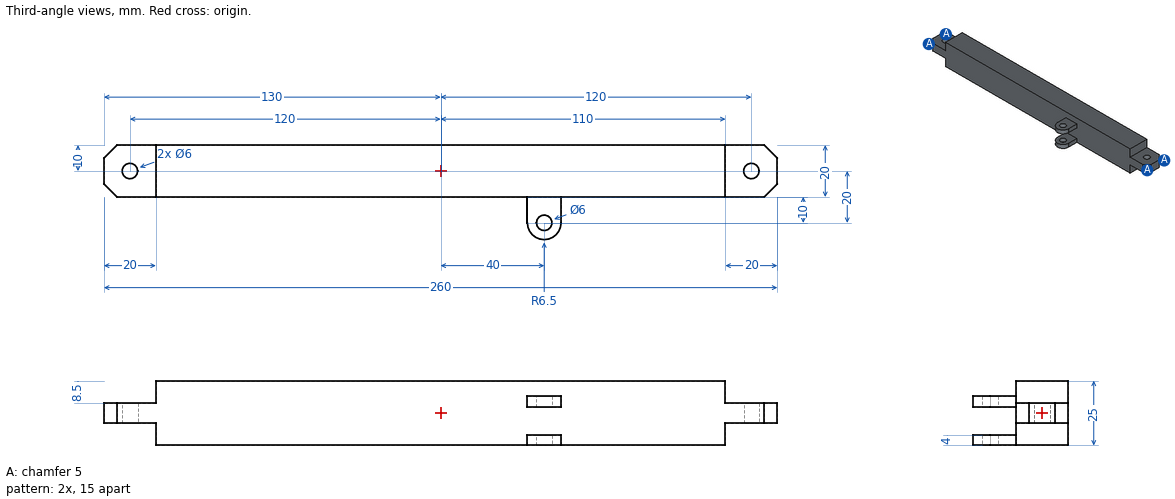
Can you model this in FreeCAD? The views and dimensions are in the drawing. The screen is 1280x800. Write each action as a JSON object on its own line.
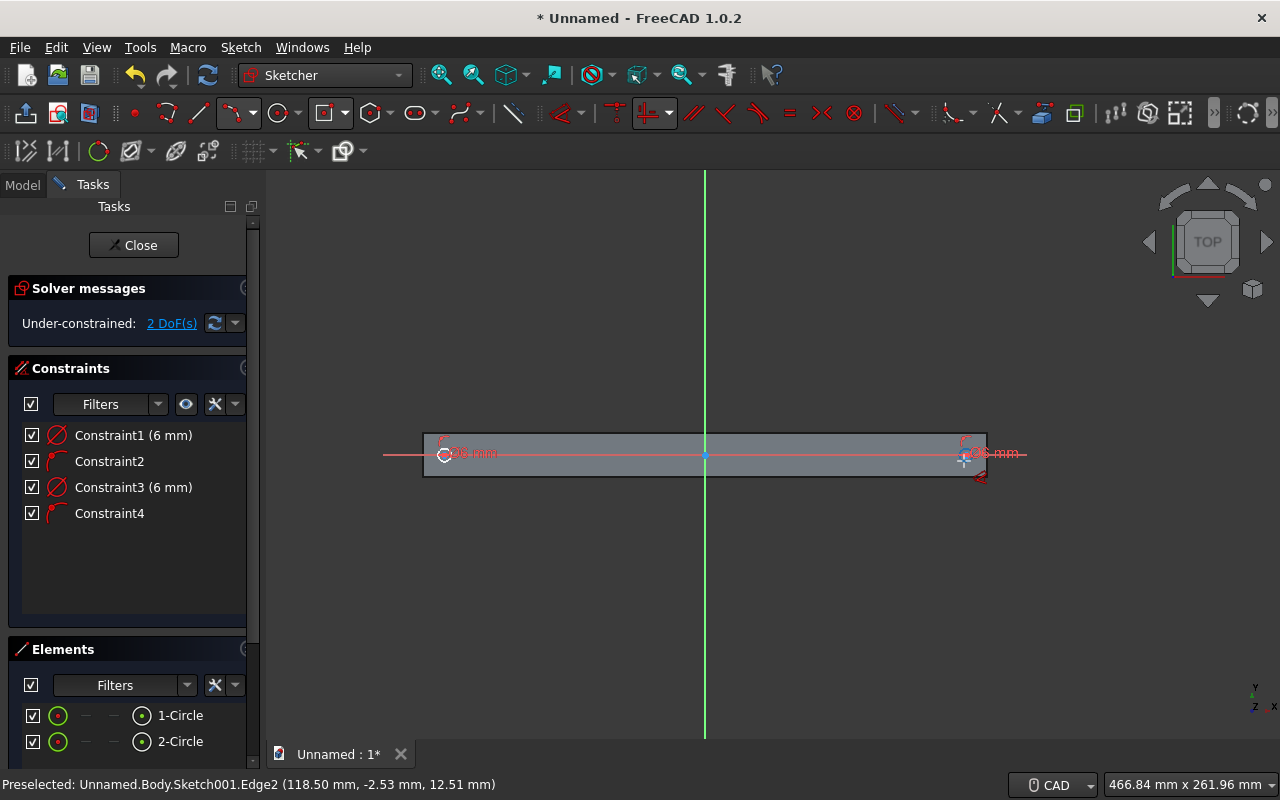
{"action": "left_click", "coordinate": [445, 455]}
{"action": "left_click", "coordinate": [575, 489]}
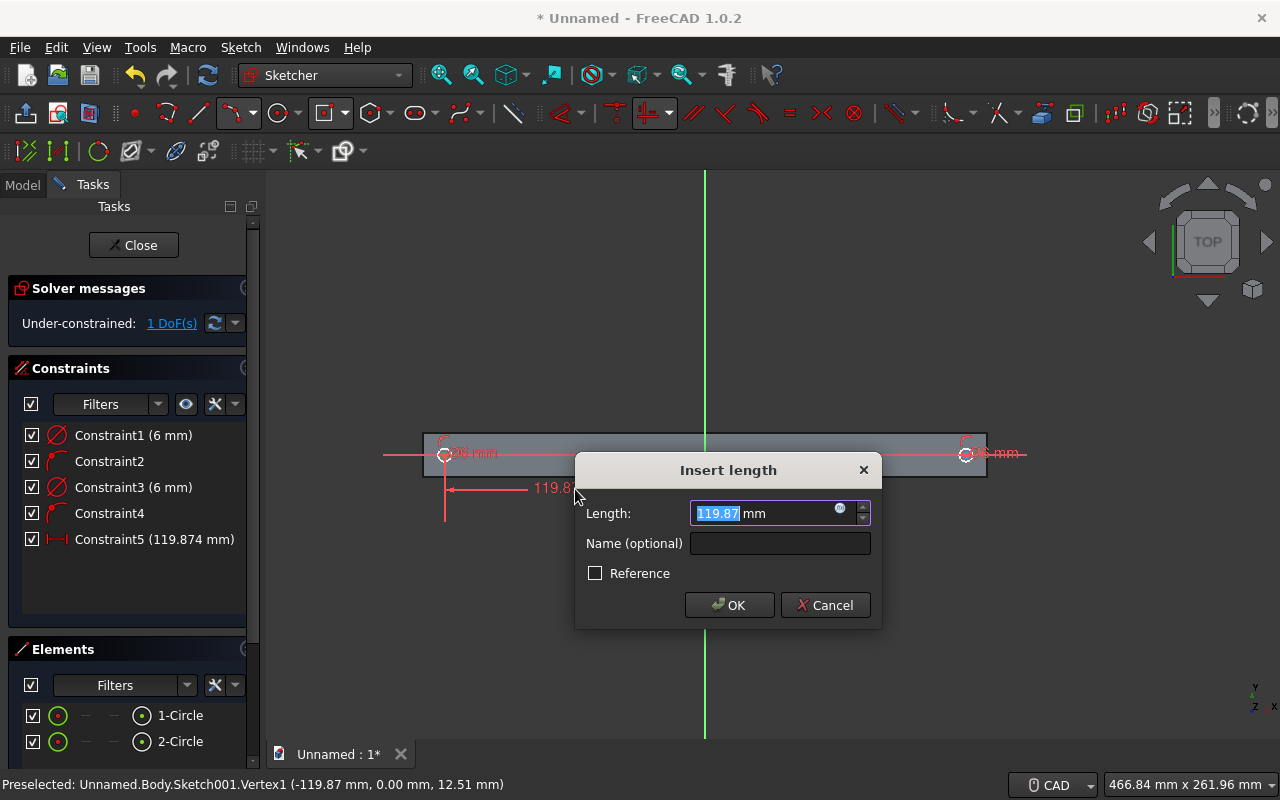
{"action": "type", "text": "120"}
{"action": "key", "text": "Return"}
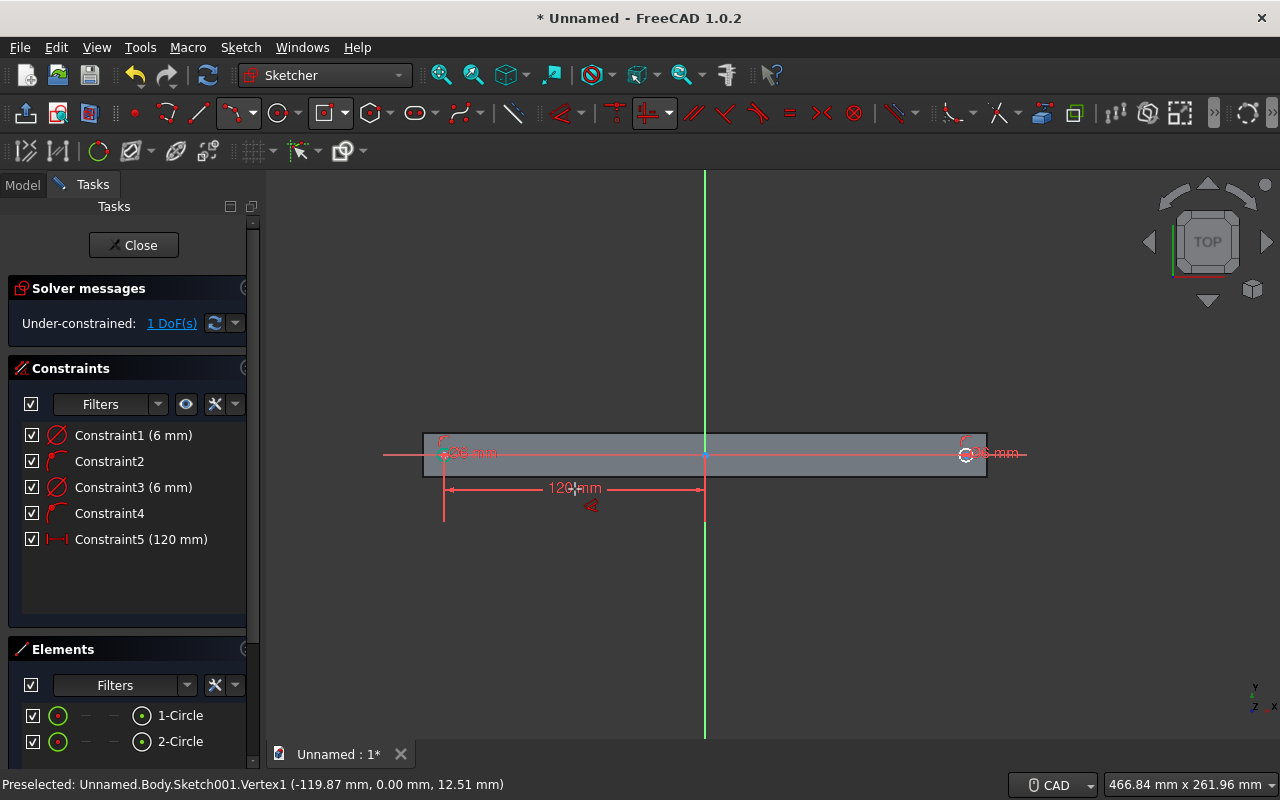
{"action": "left_click", "coordinate": [966, 455]}
{"action": "left_click", "coordinate": [836, 489]}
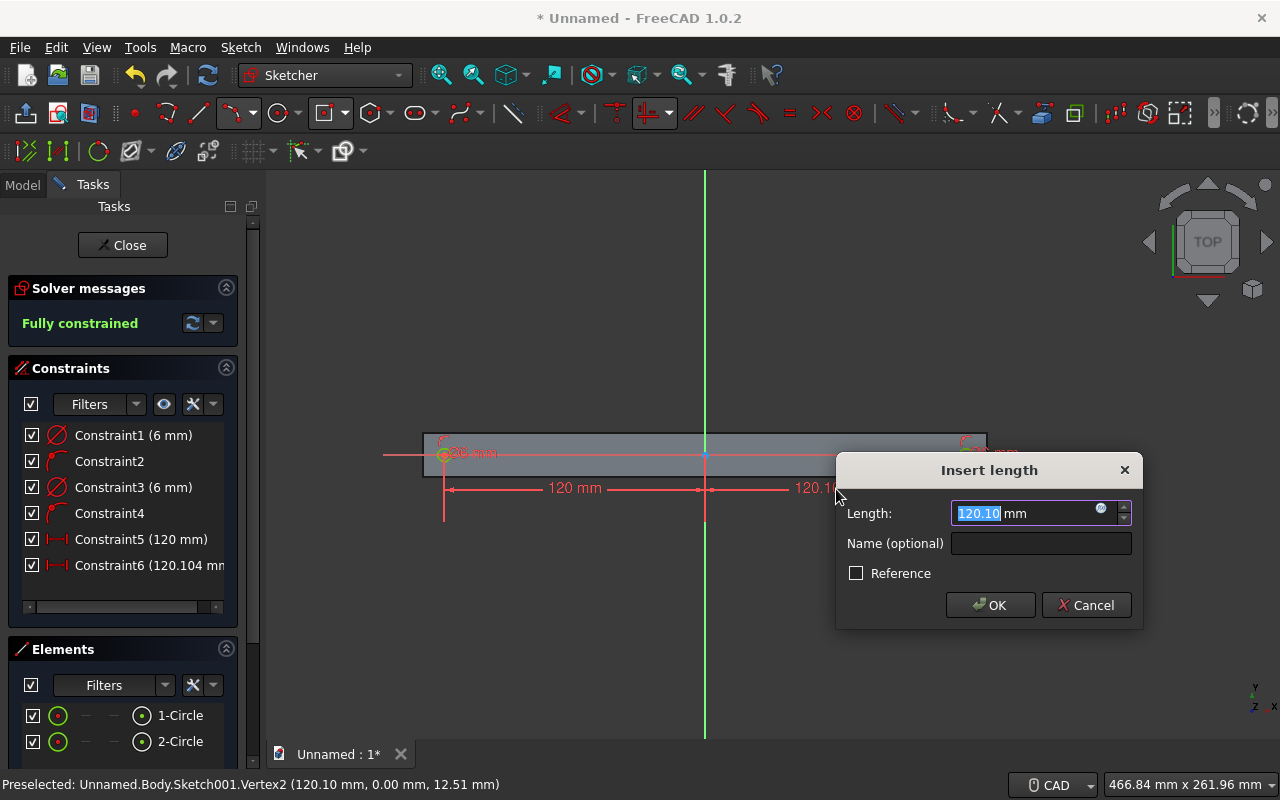
{"action": "type", "text": "120"}
{"action": "key", "text": "Return"}
{"action": "key", "text": "Escape"}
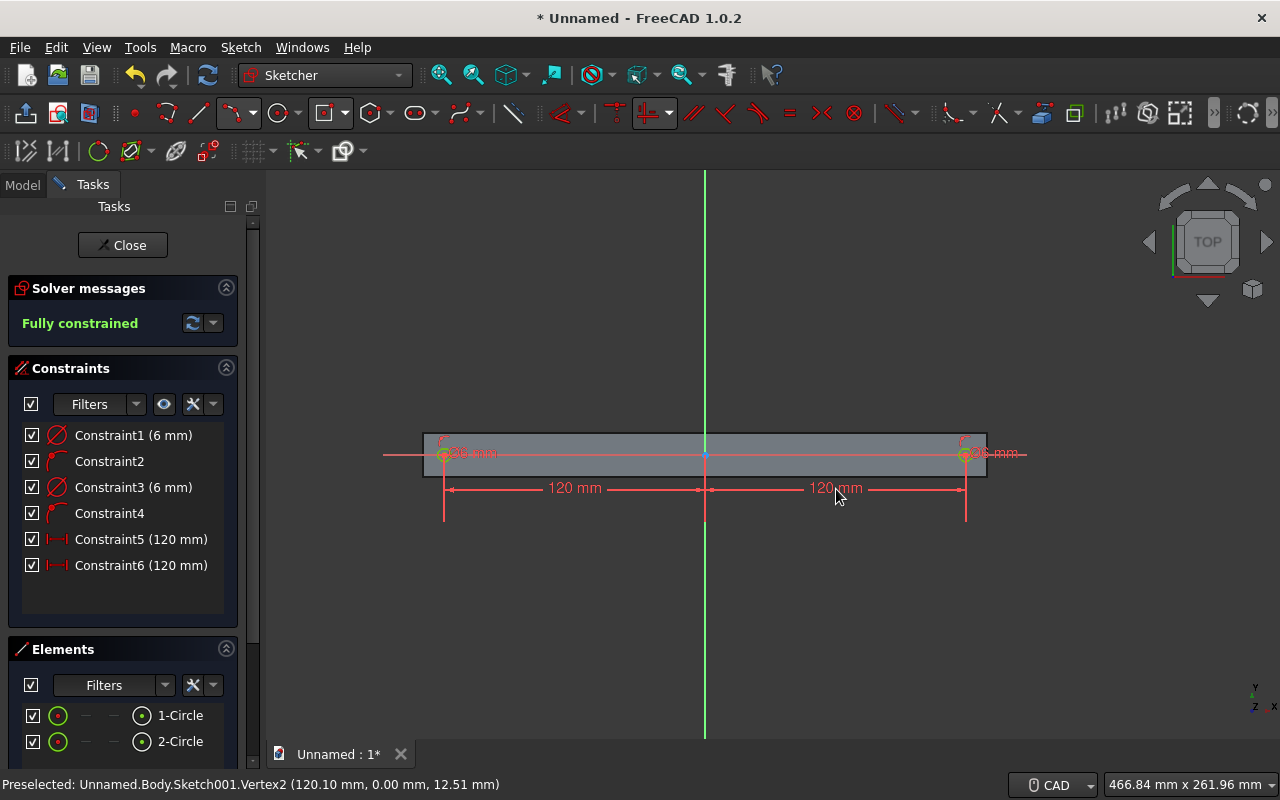
{"action": "left_click", "coordinate": [123, 245]}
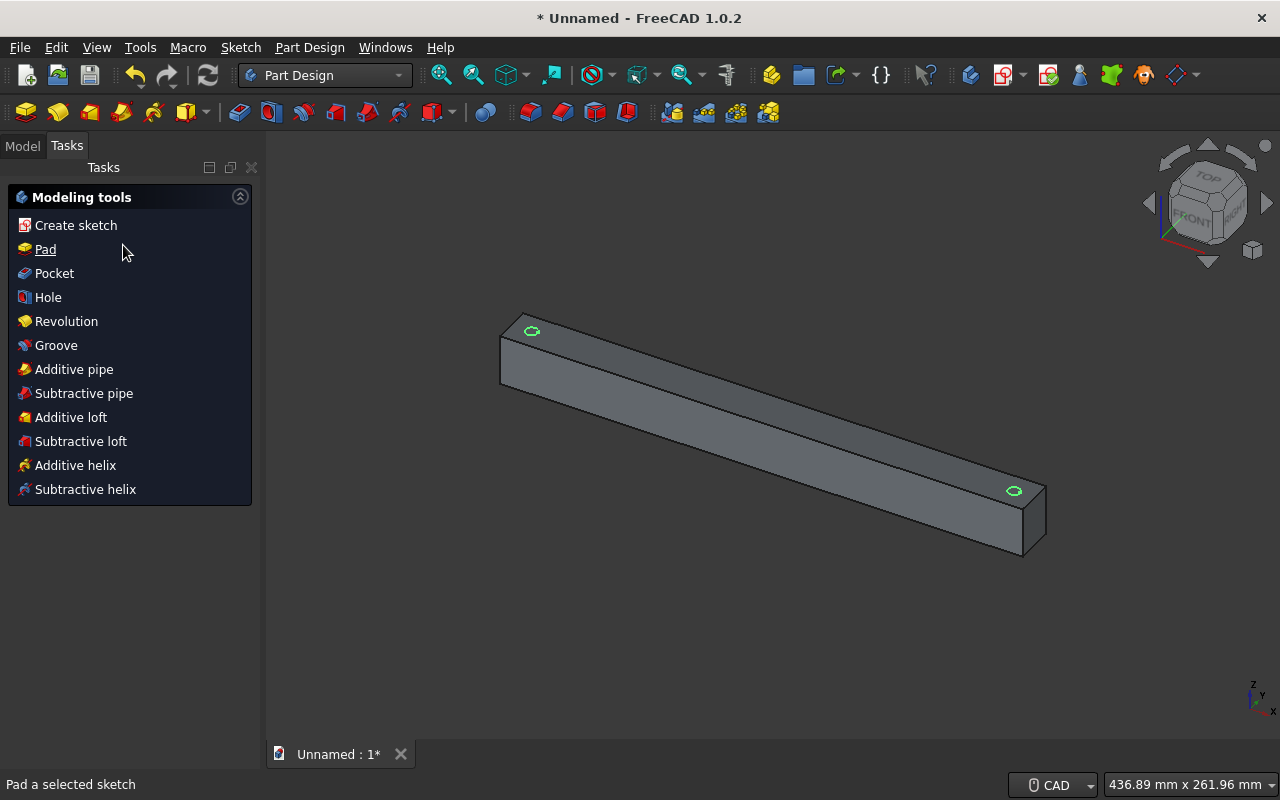
{"action": "left_click", "coordinate": [240, 112]}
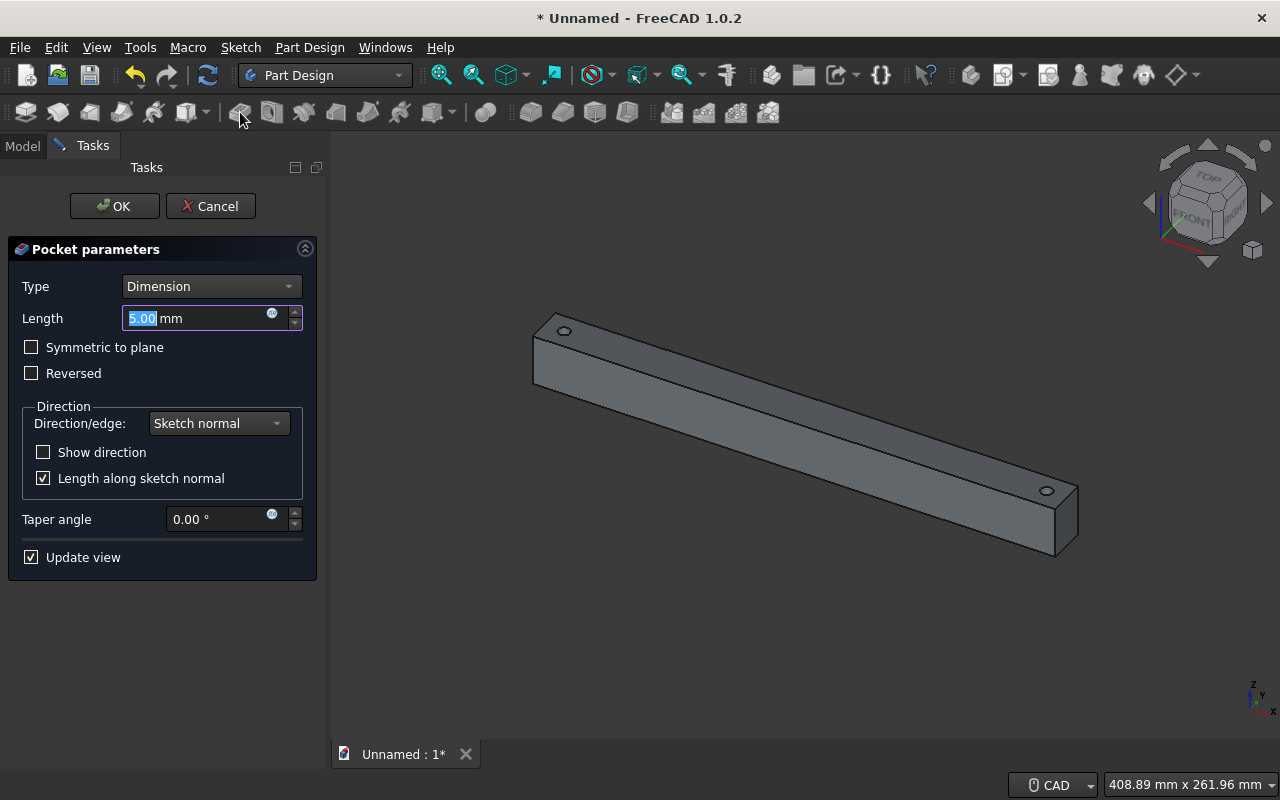
{"action": "left_click", "coordinate": [212, 286]}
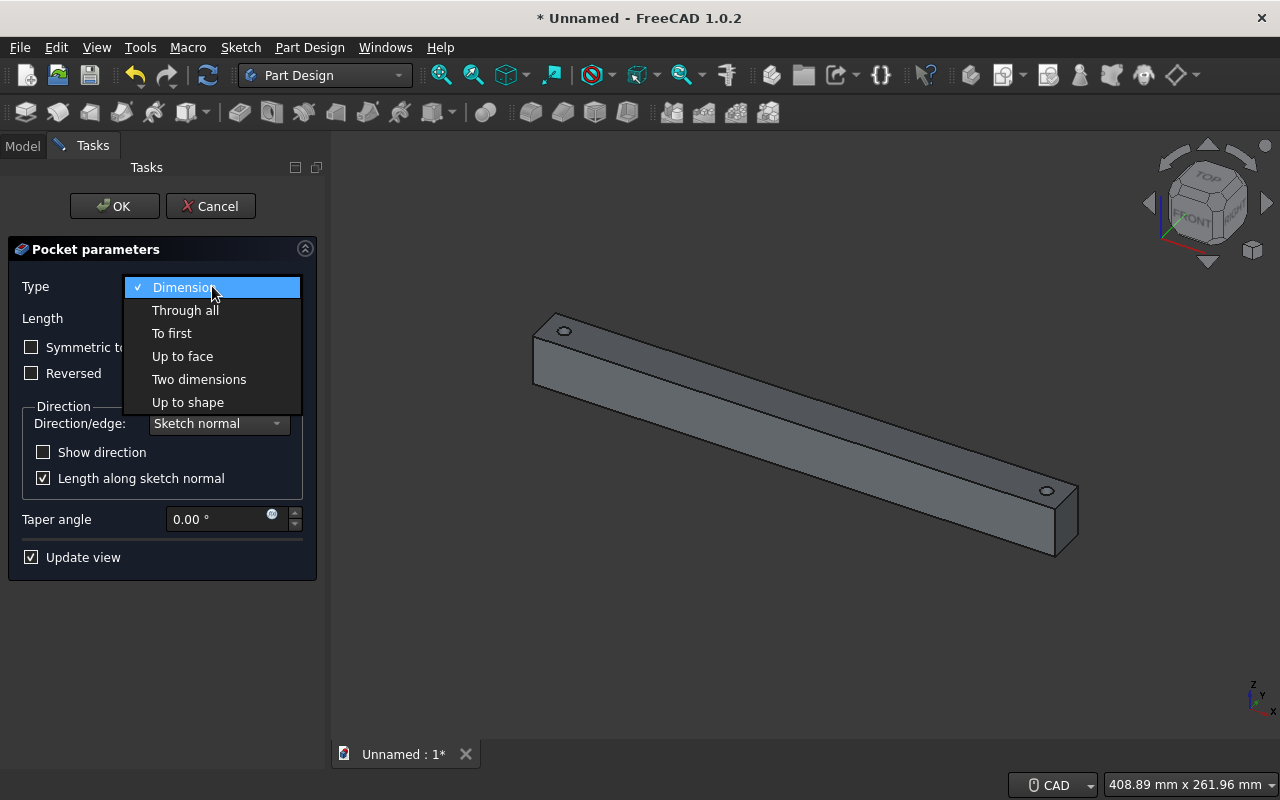
{"action": "left_click", "coordinate": [212, 310]}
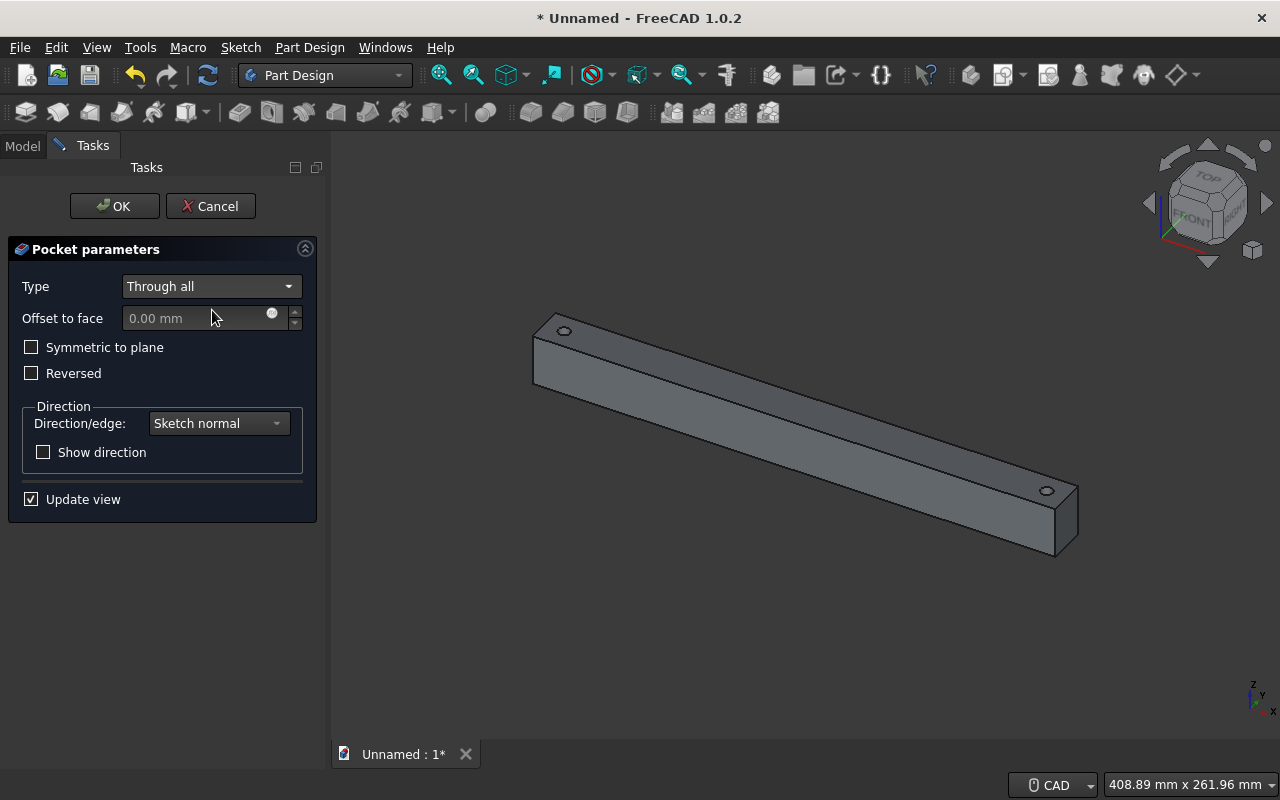
{"action": "left_click", "coordinate": [115, 206]}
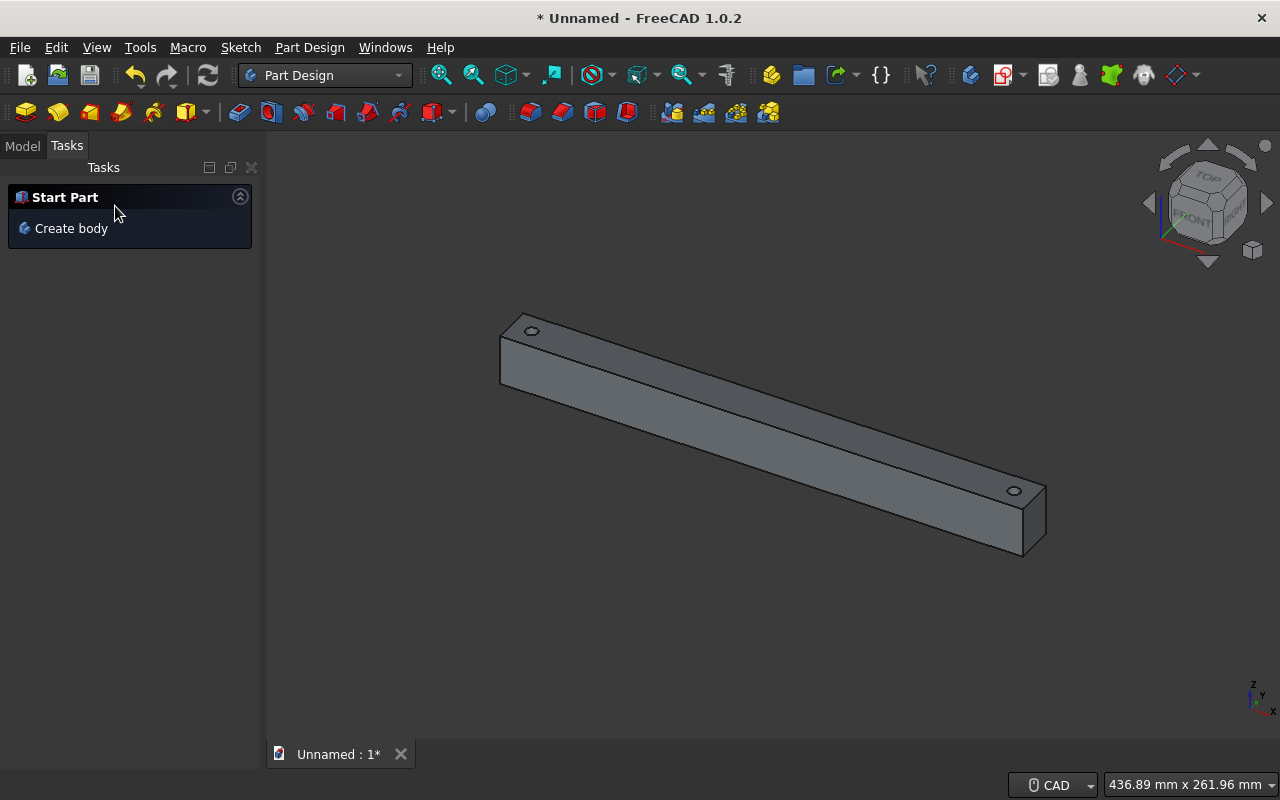
{"action": "left_click", "coordinate": [922, 460]}